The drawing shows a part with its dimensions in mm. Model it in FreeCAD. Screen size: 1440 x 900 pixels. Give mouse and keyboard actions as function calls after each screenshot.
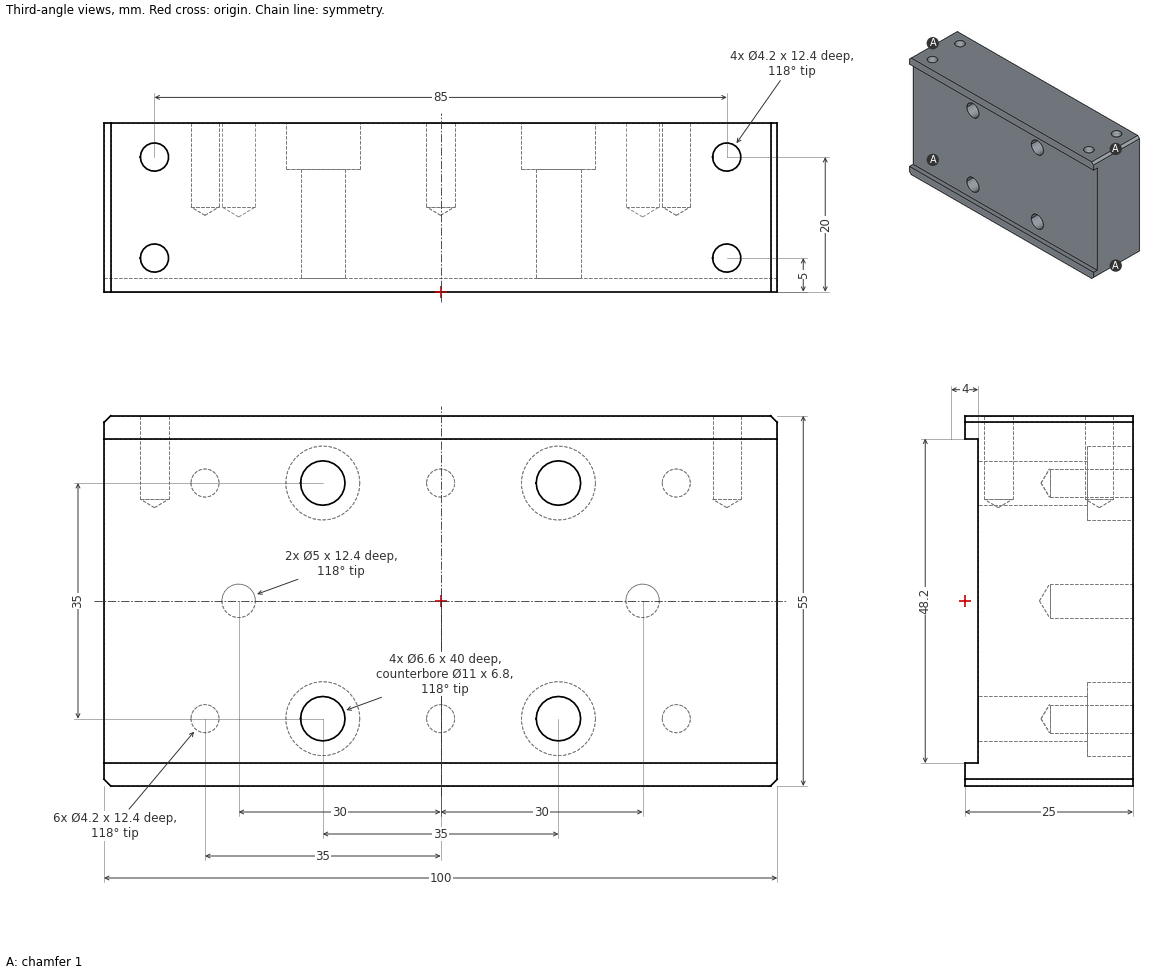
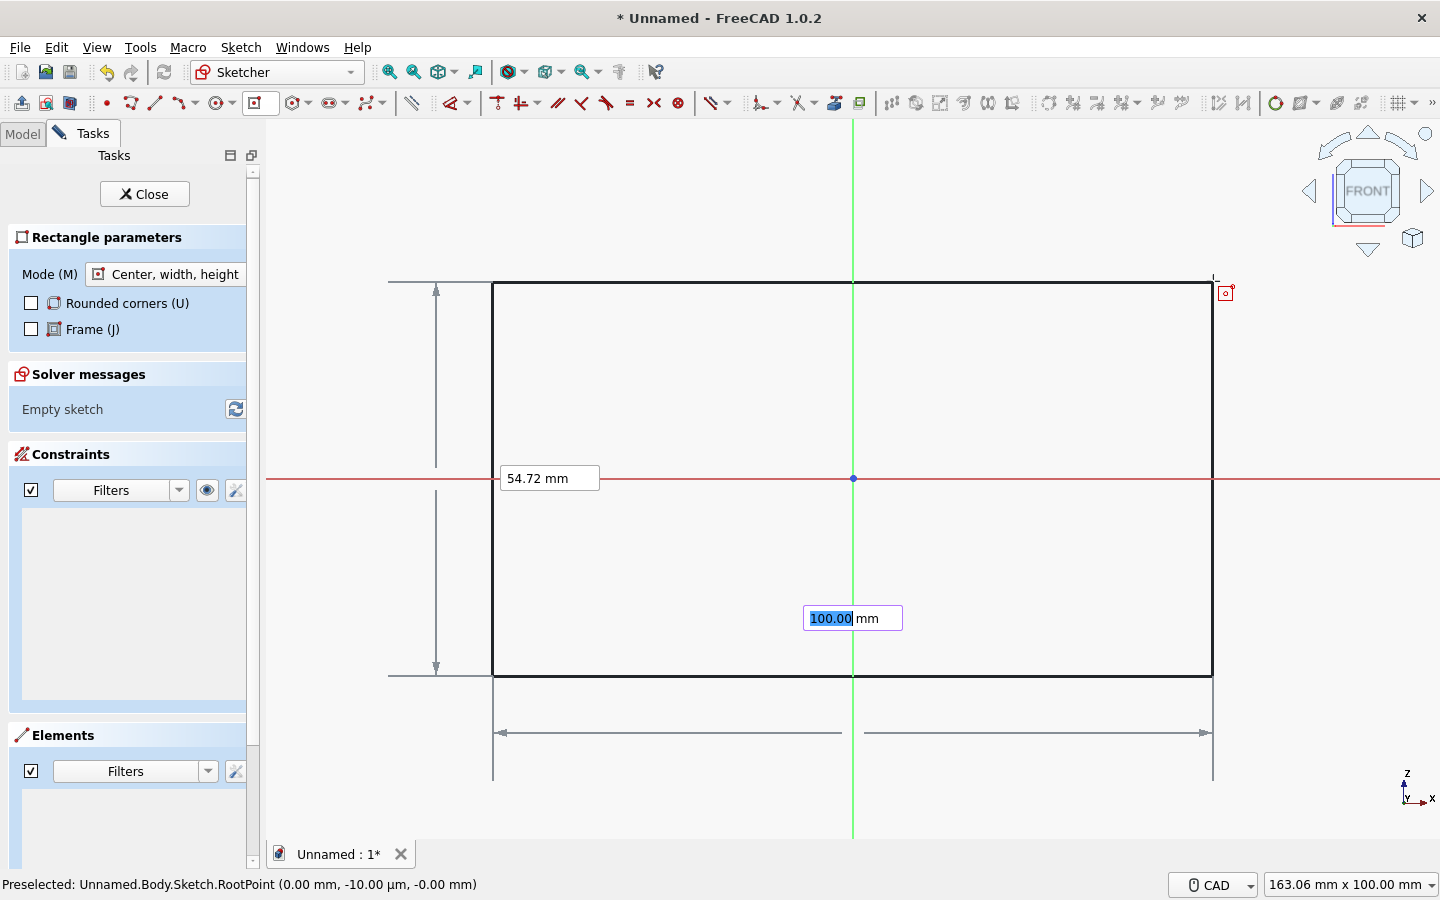
text(100)
key(Tab)
text(55)
key(Return)
key(Escape)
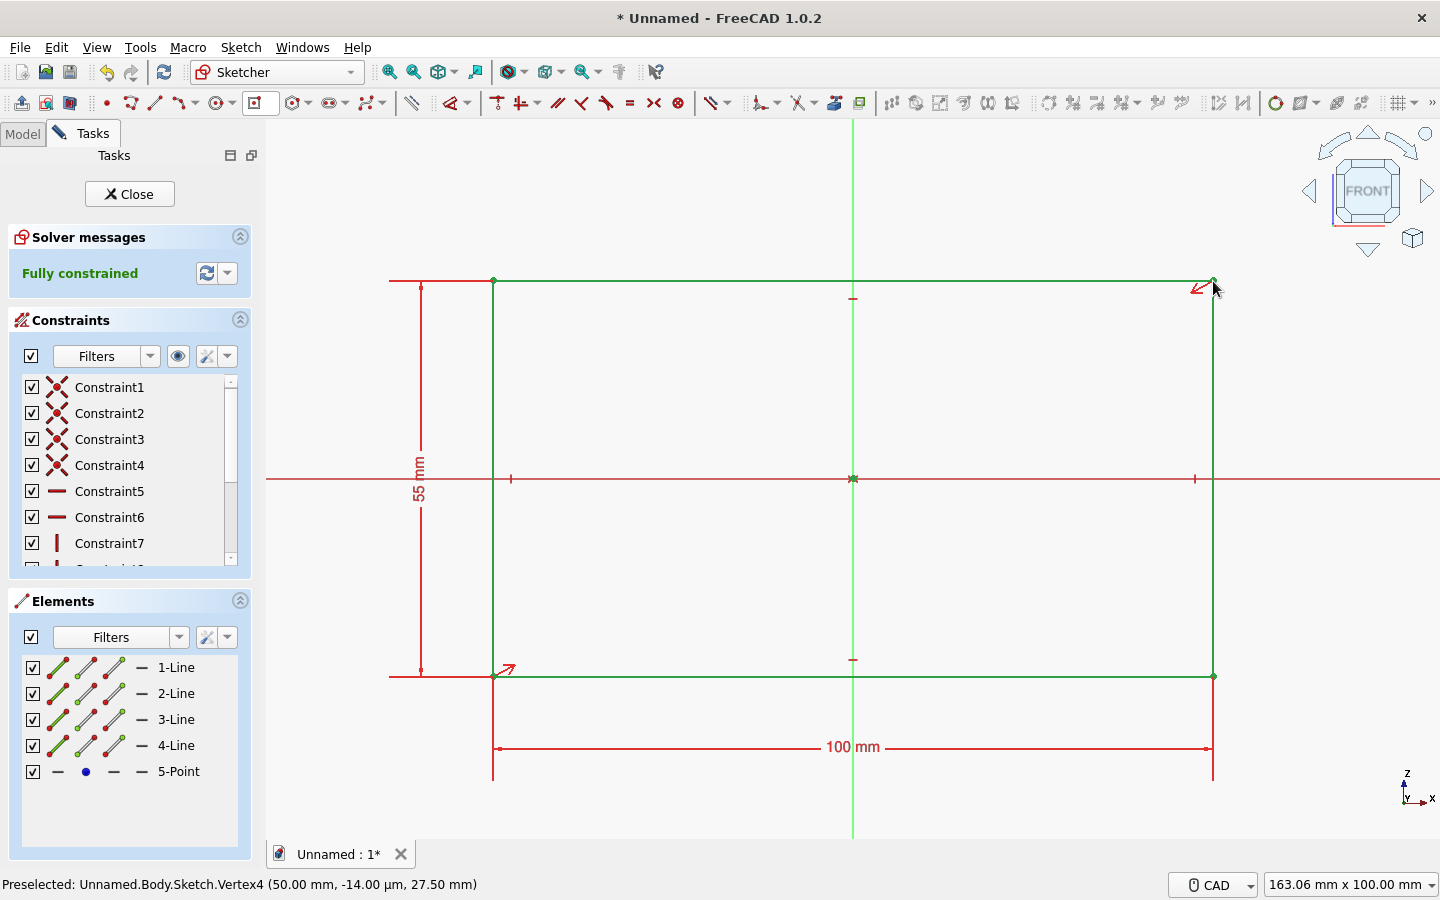
click(130, 194)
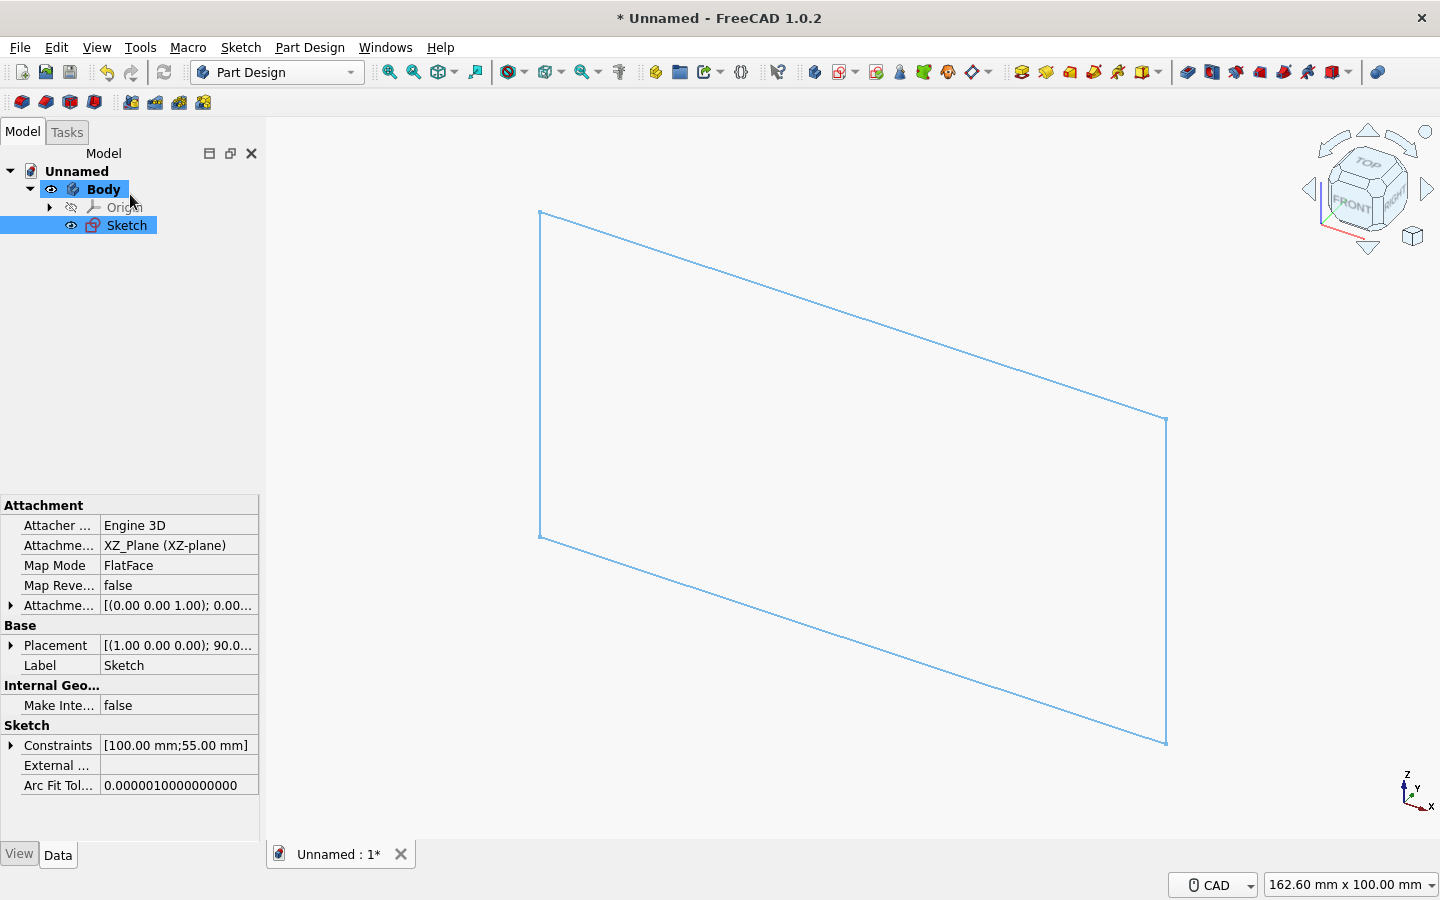
click(1022, 72)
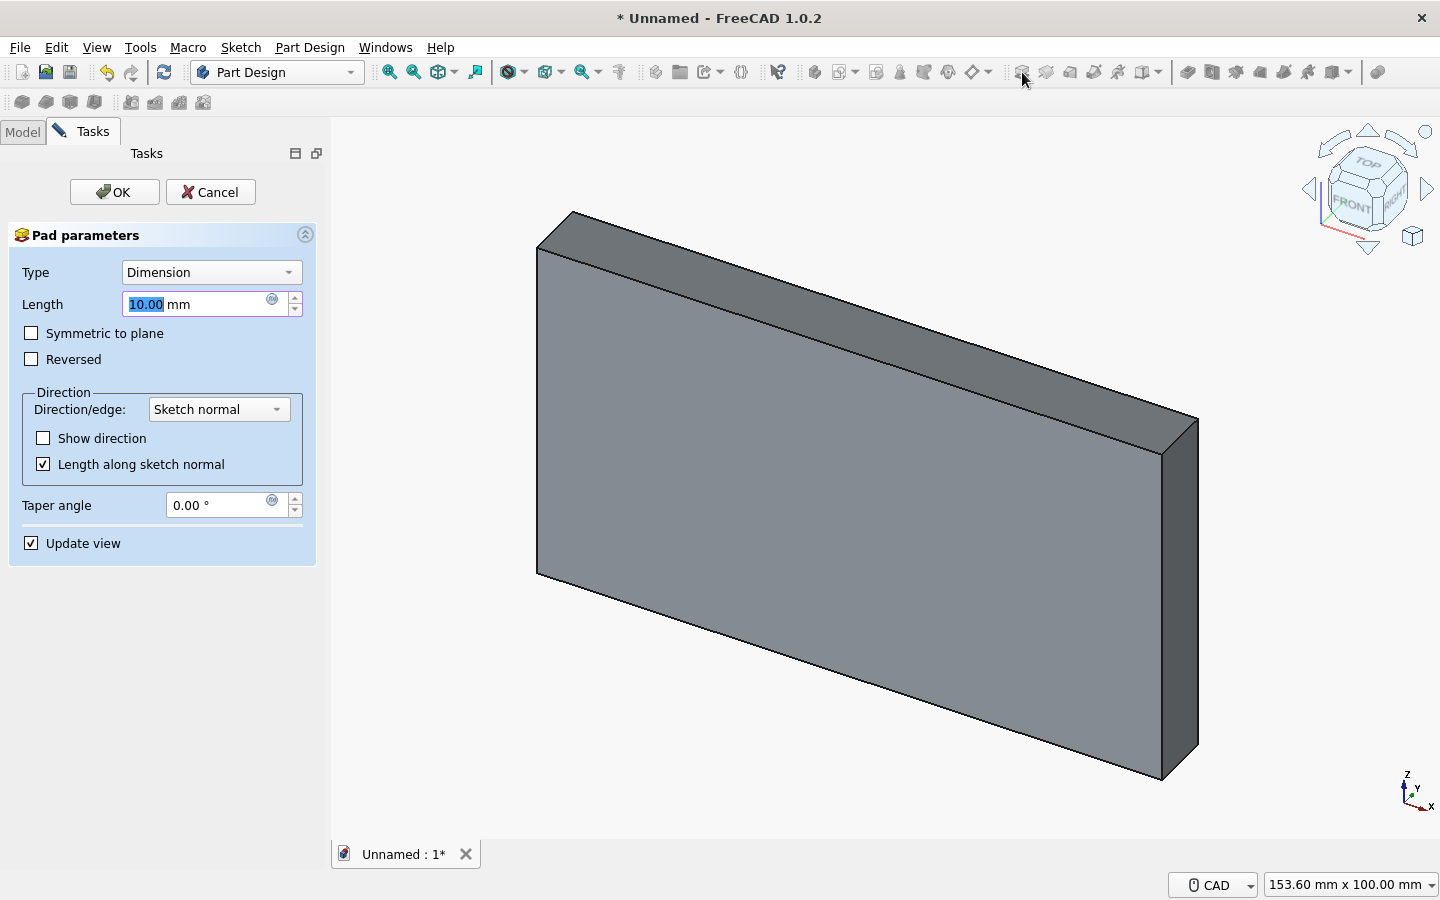
text(25)
key(Tab)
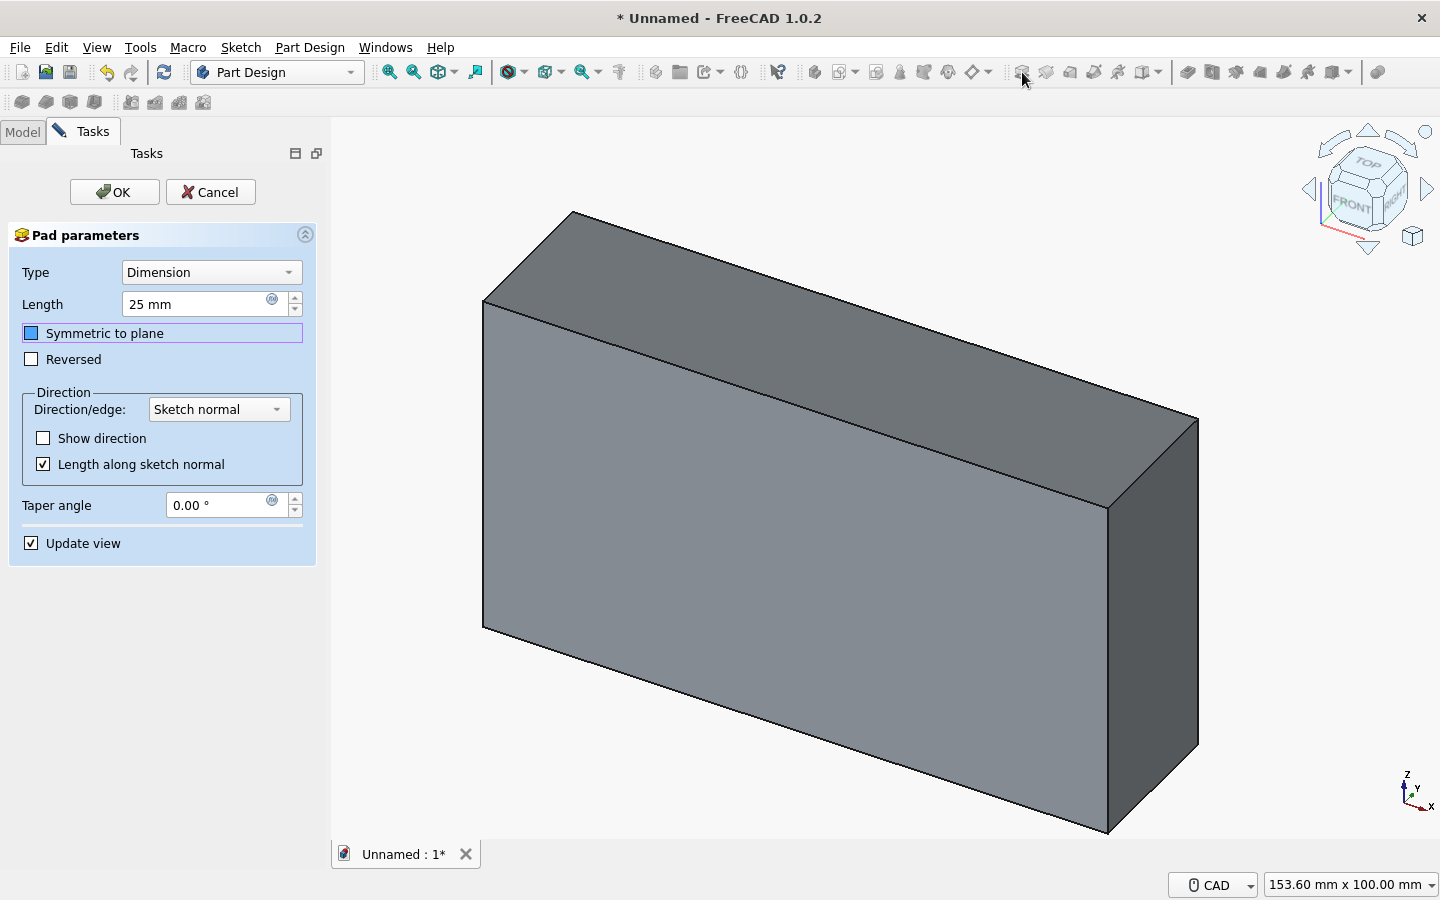
click(30, 359)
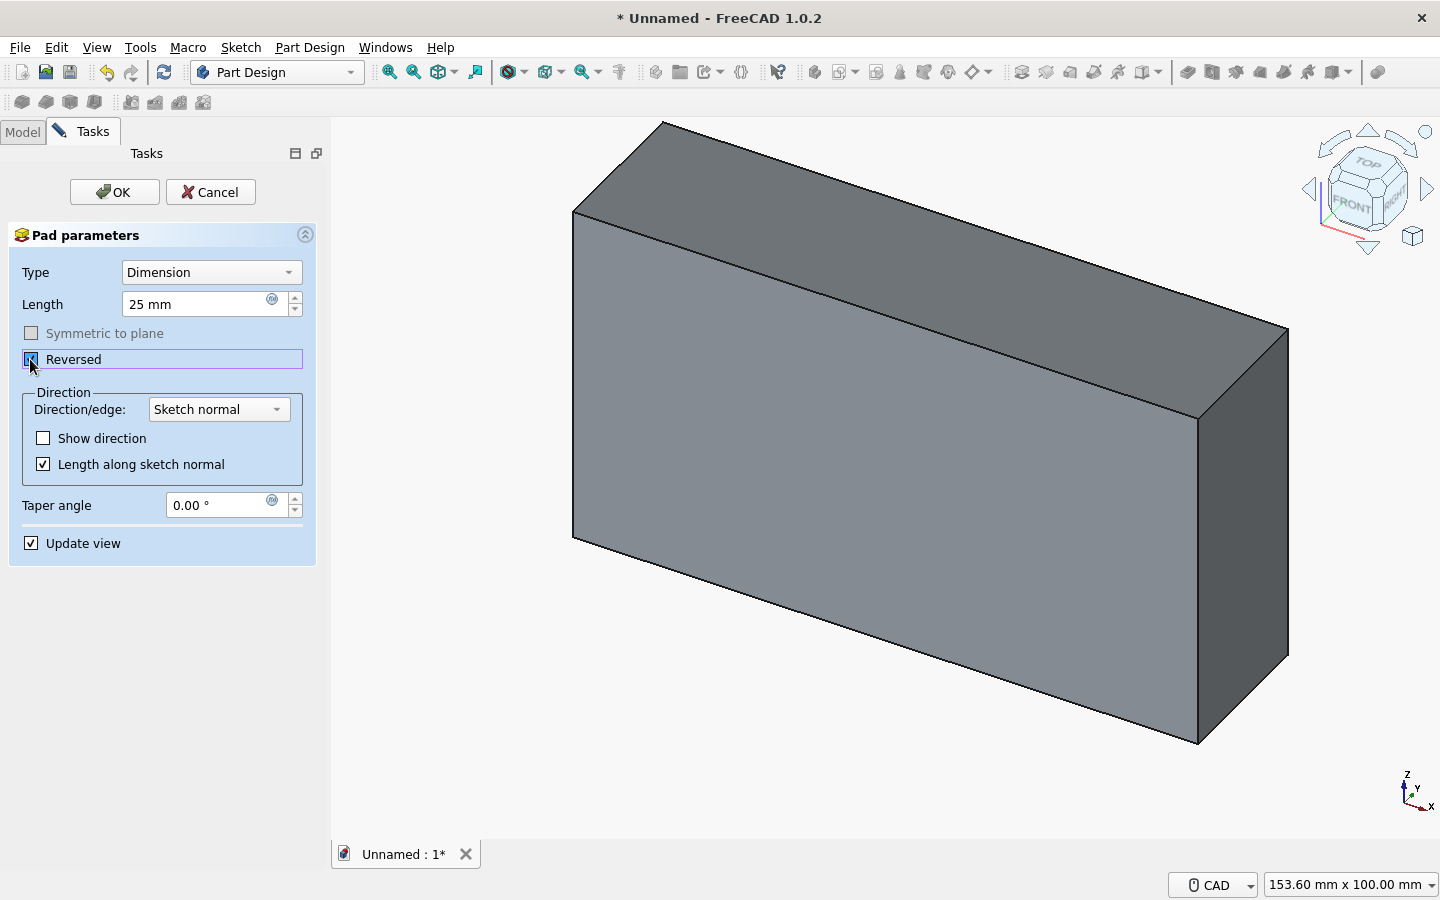
click(115, 192)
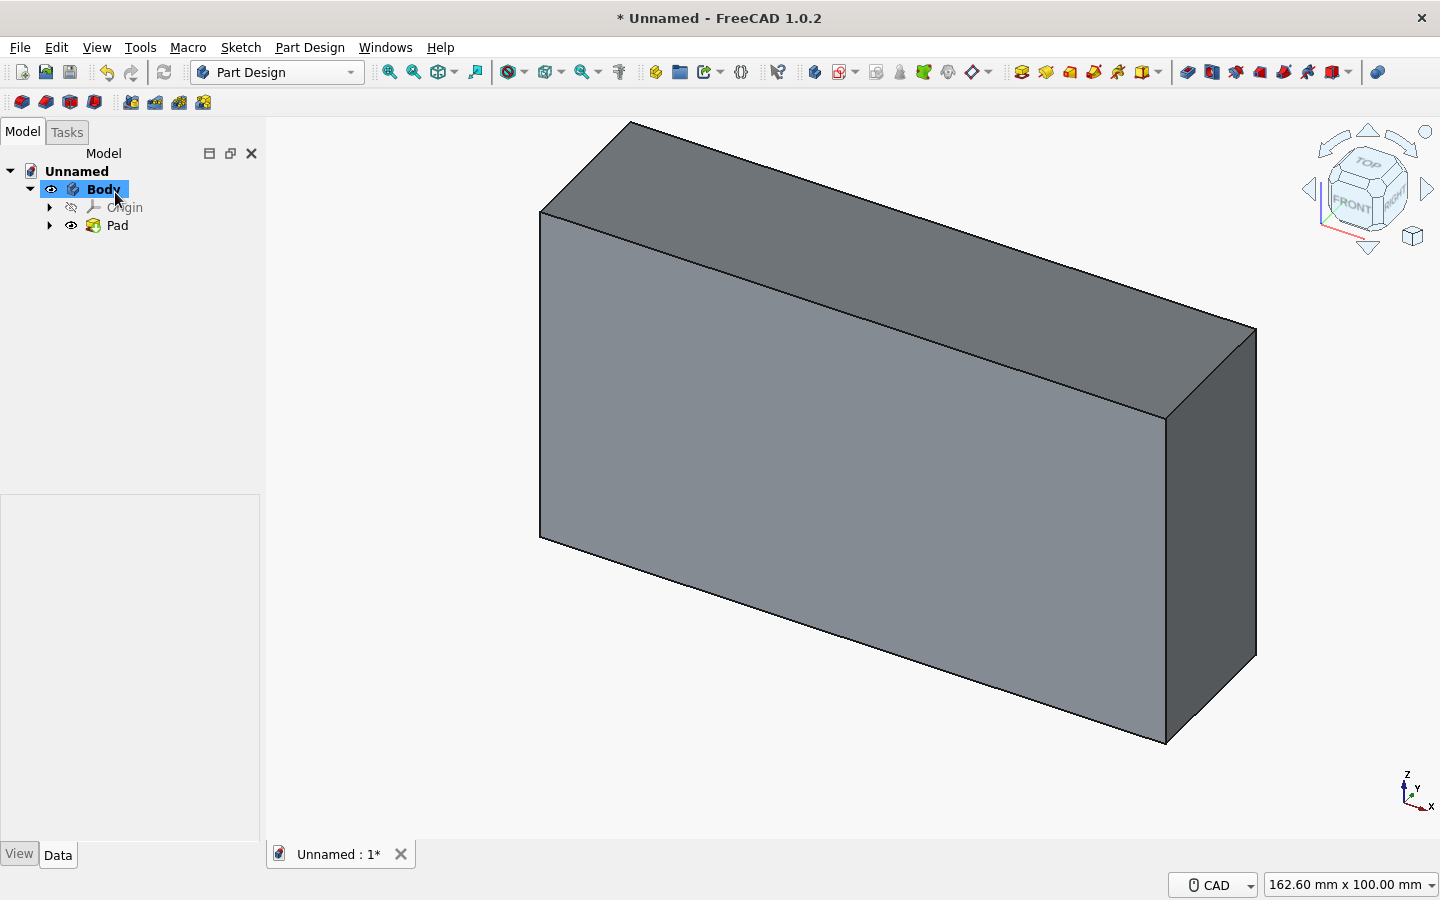
click(1211, 536)